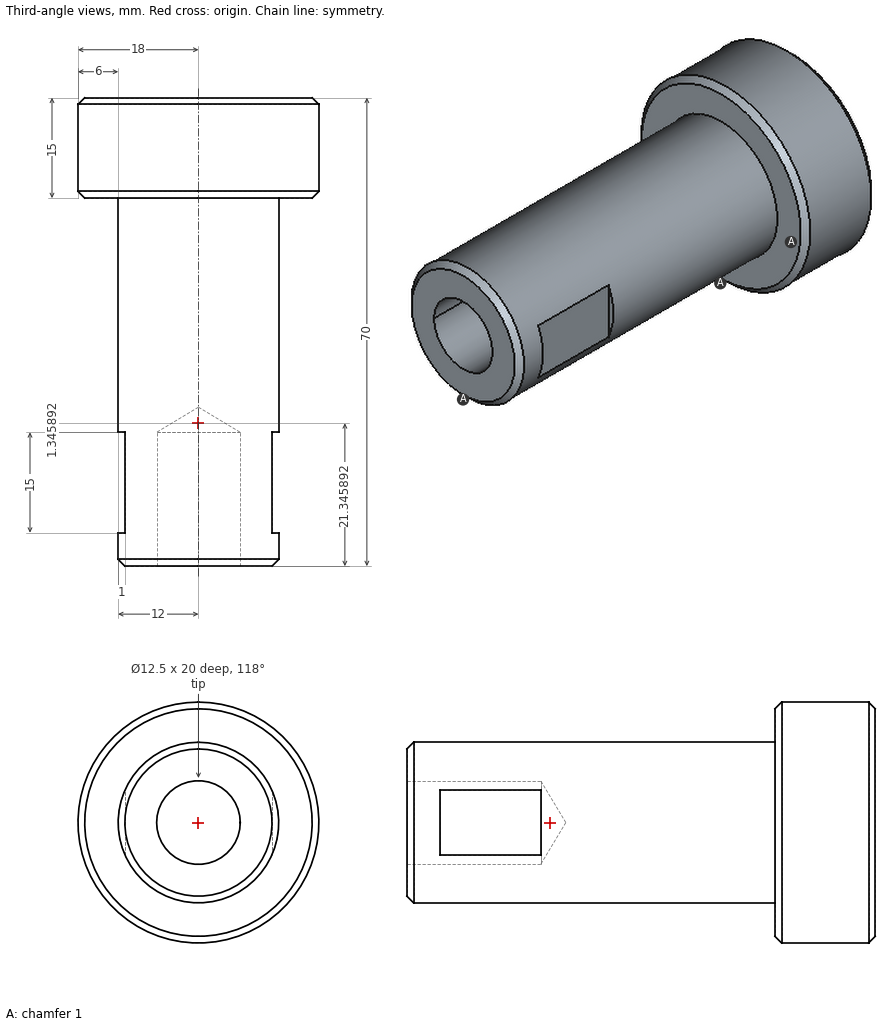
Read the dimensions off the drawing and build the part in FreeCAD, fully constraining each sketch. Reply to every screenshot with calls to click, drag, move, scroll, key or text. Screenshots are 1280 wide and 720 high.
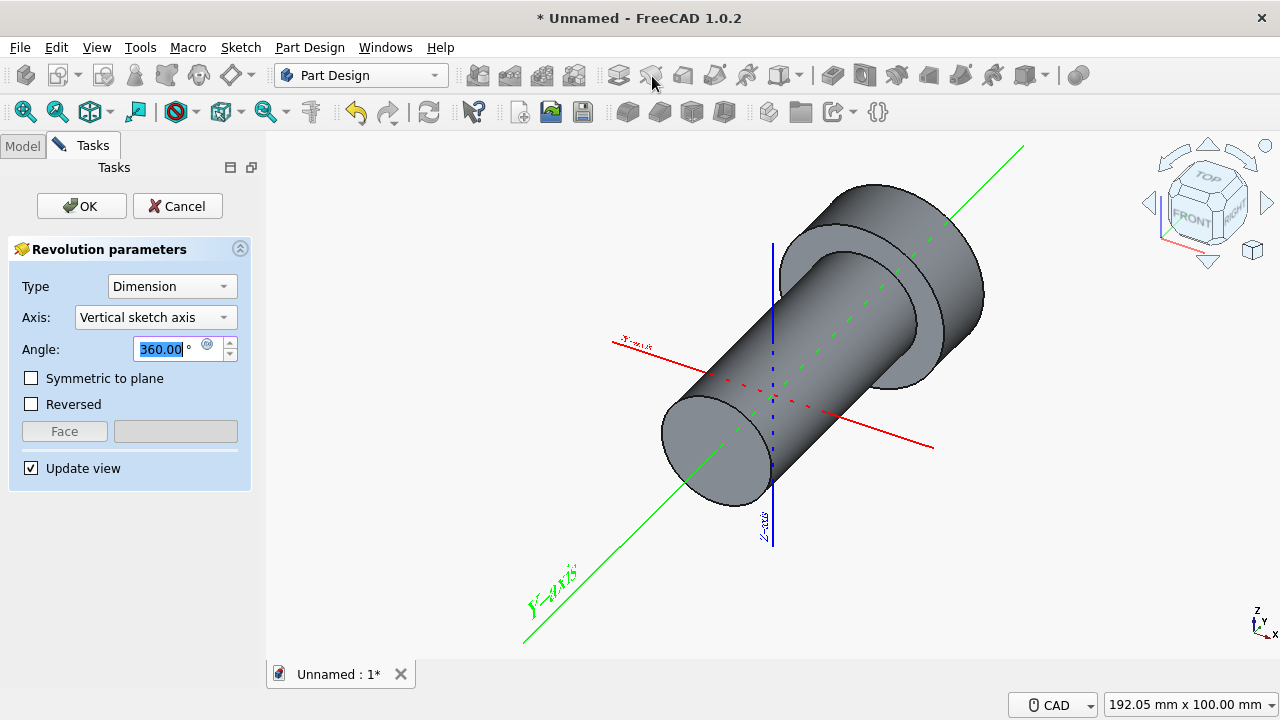
click(82, 206)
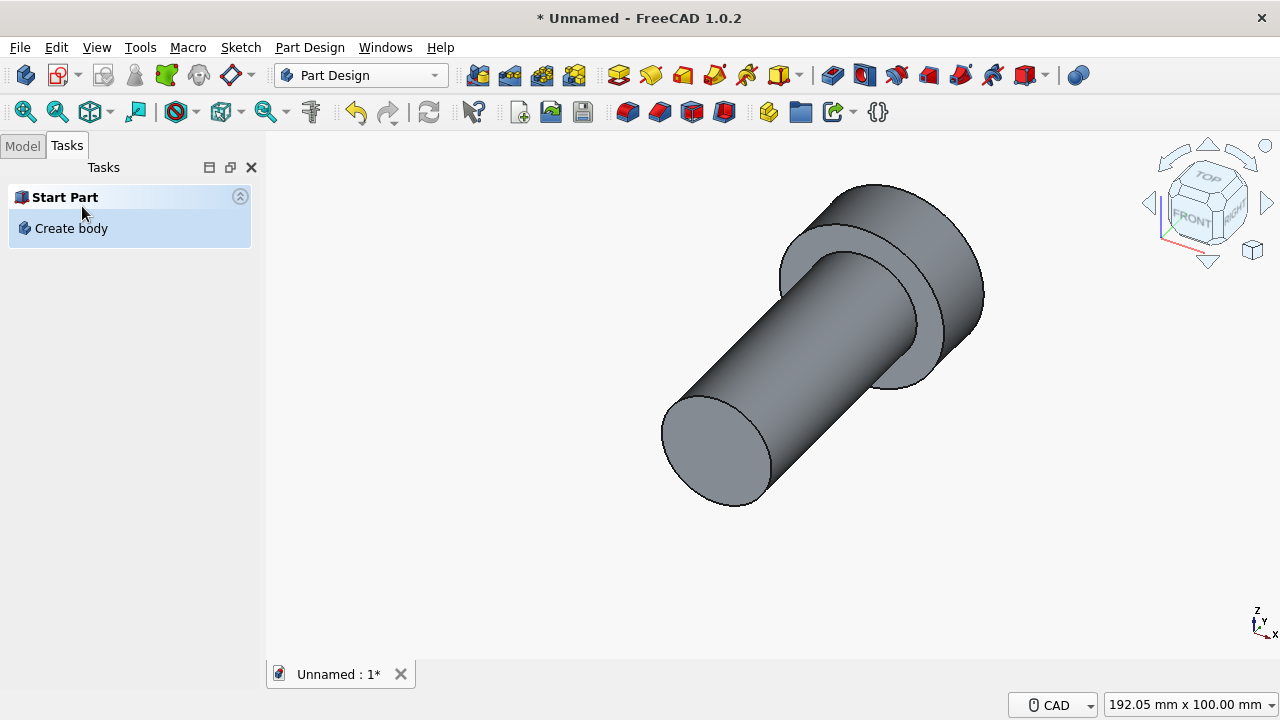
click(772, 468)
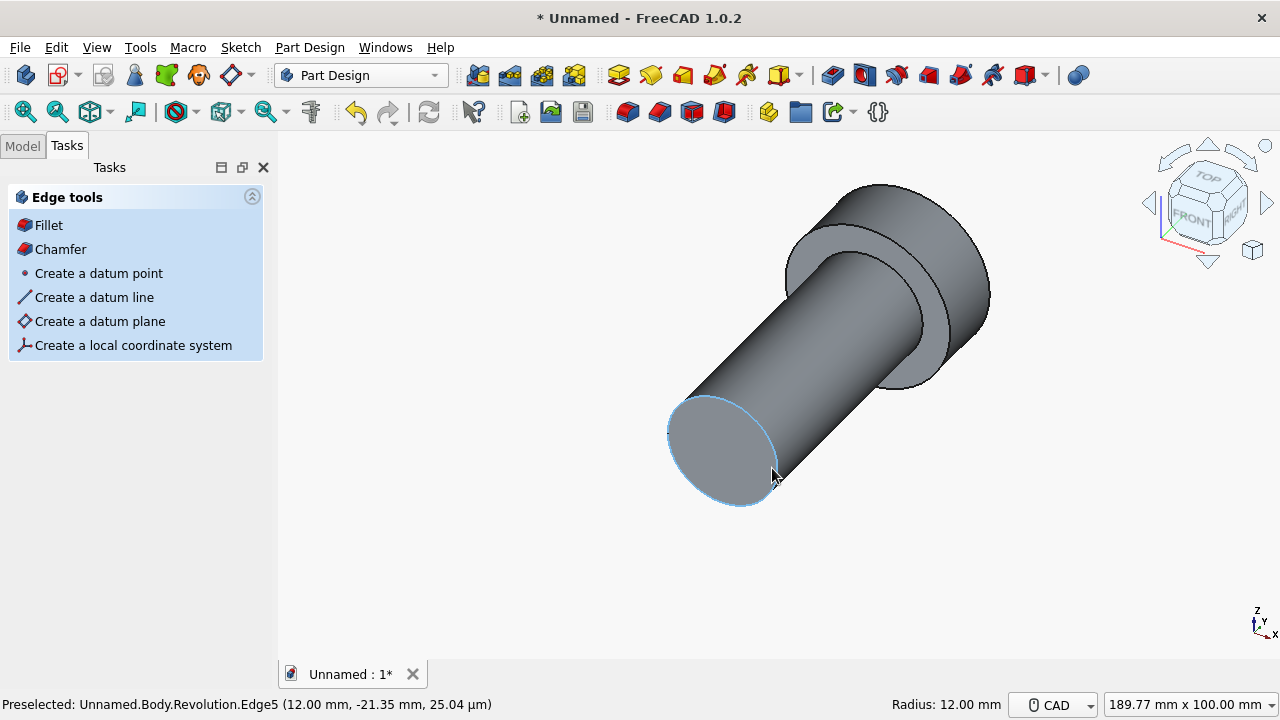
click(950, 333, ctrl)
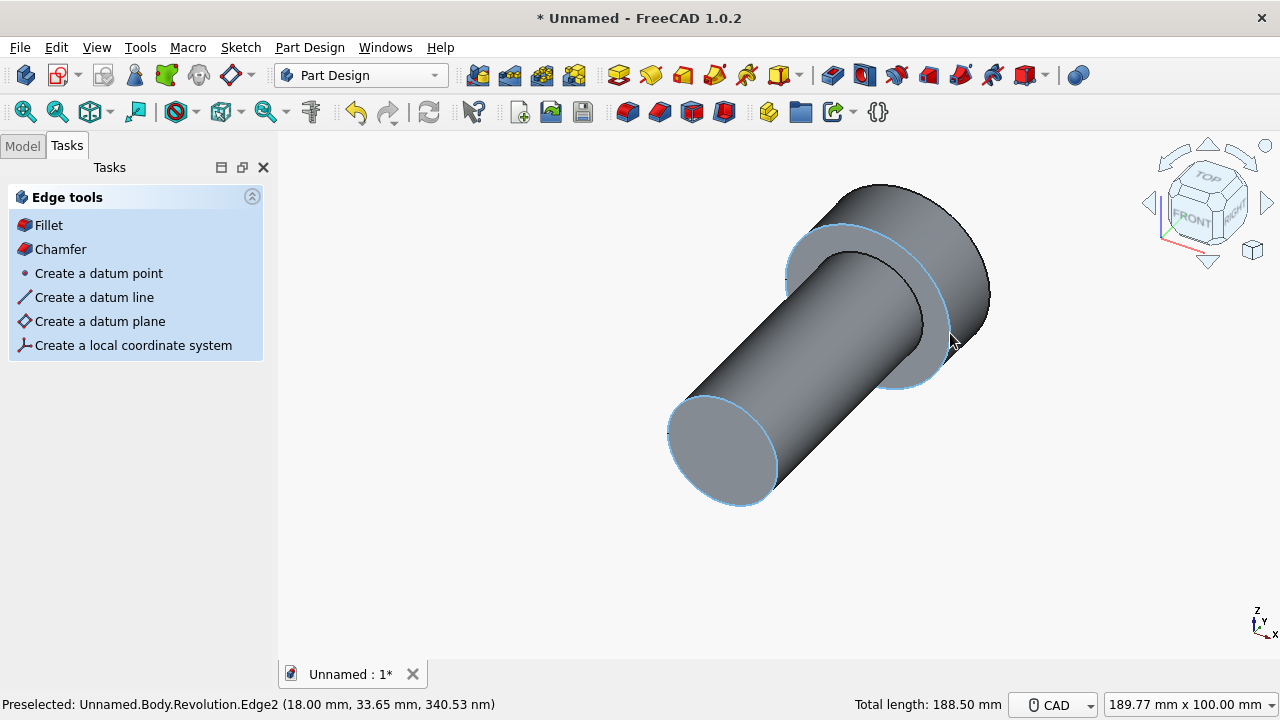
key(0)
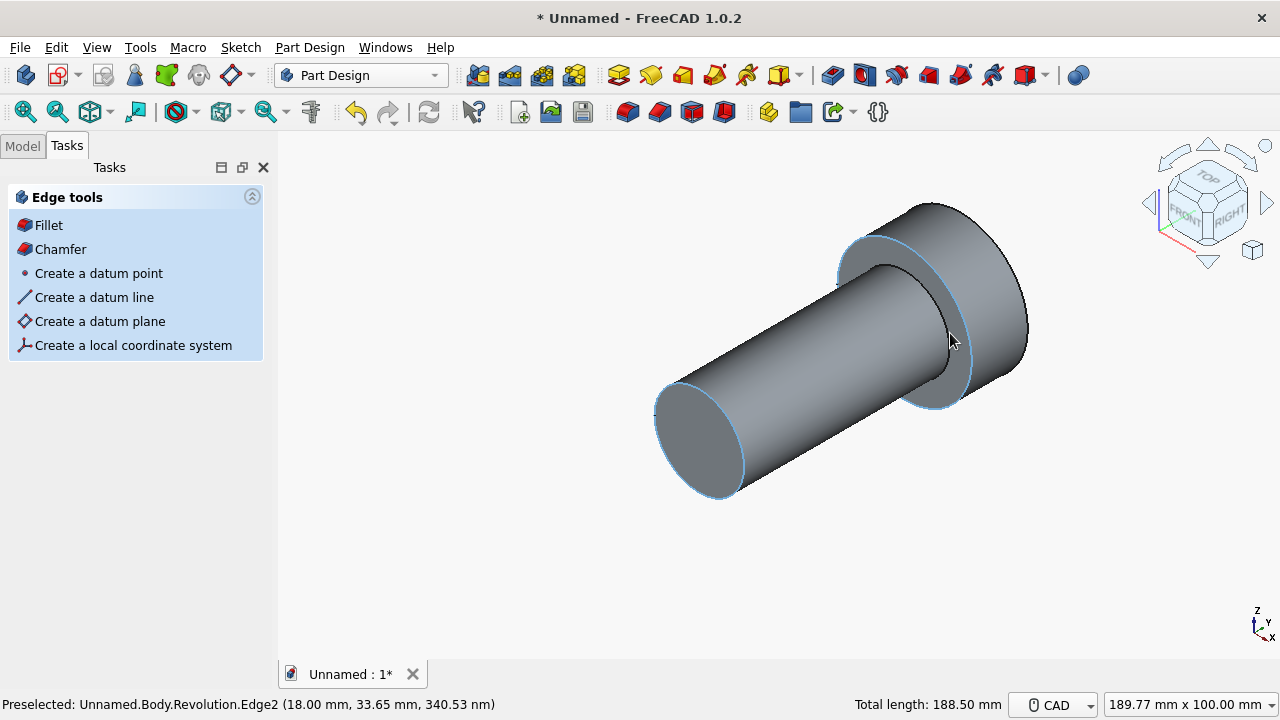
key(2)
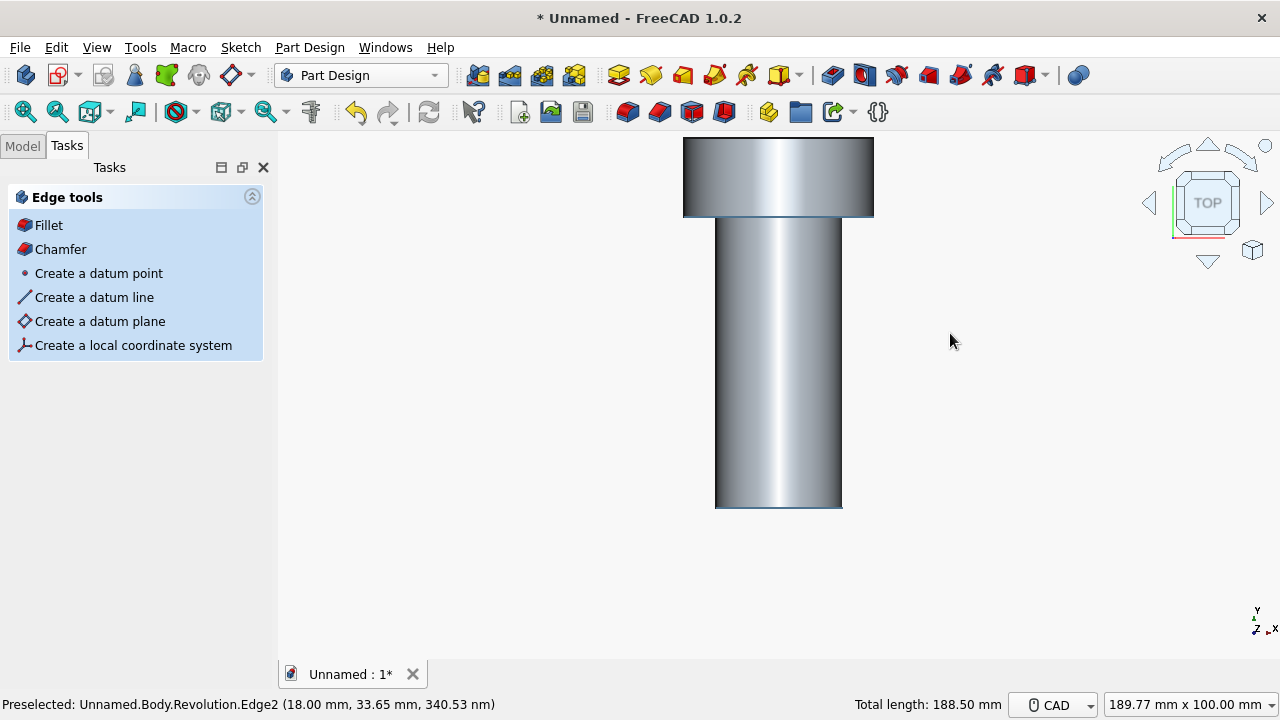
key(1)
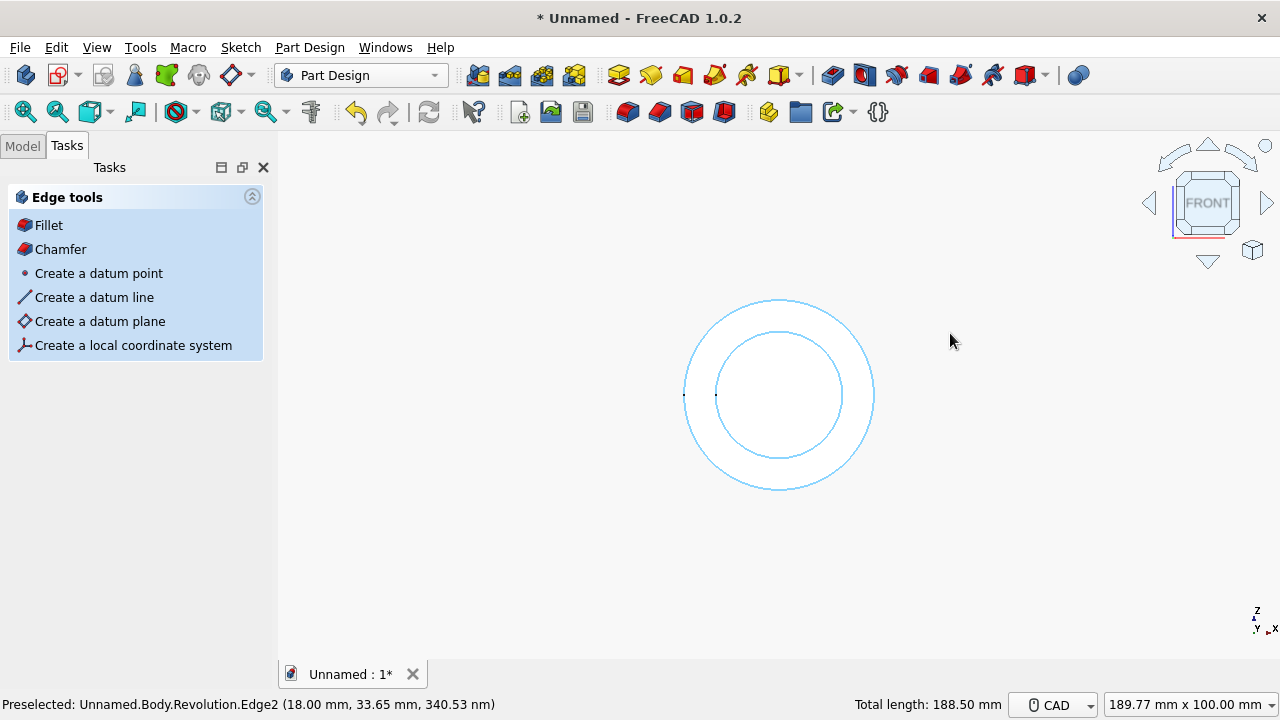
click(26, 112)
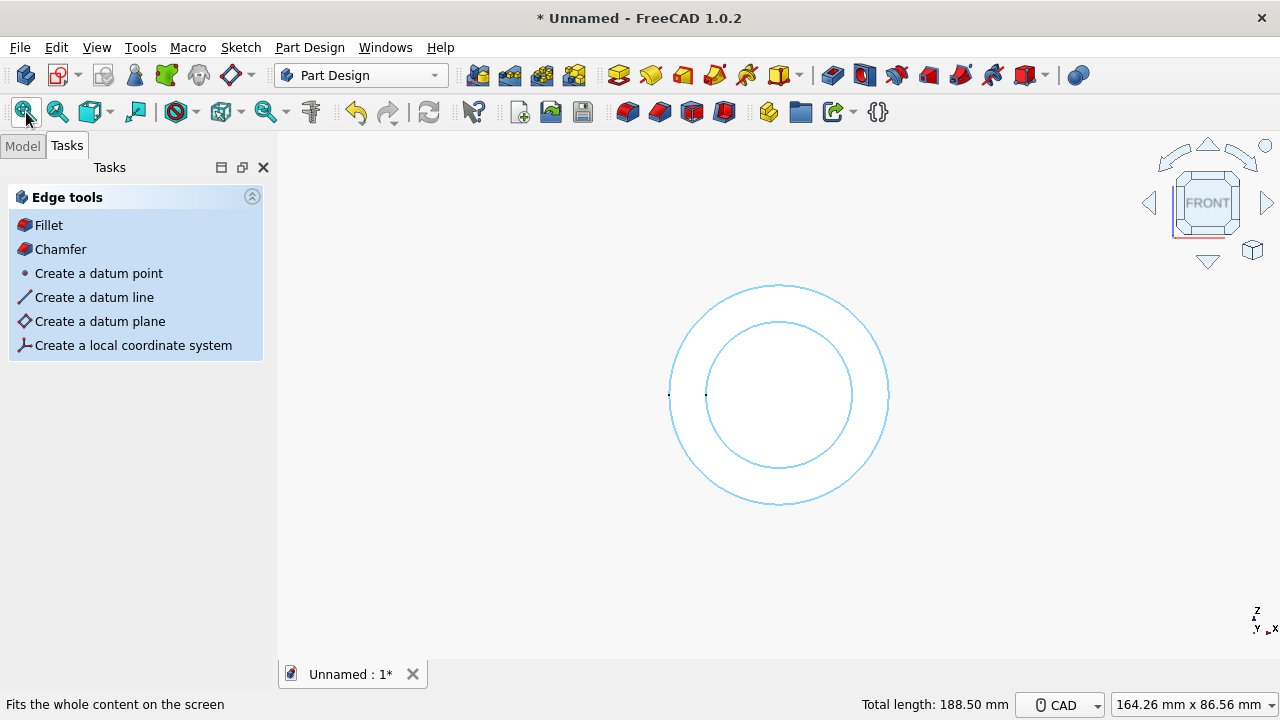
key(3)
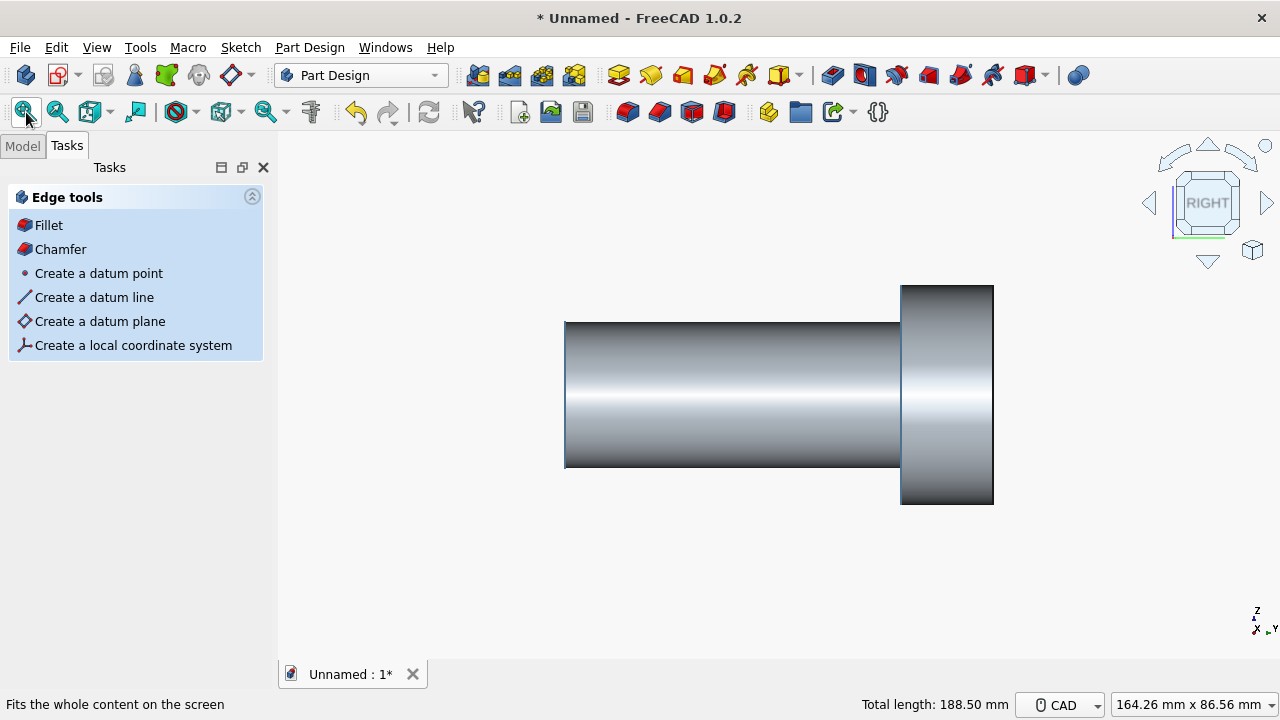
click(26, 112)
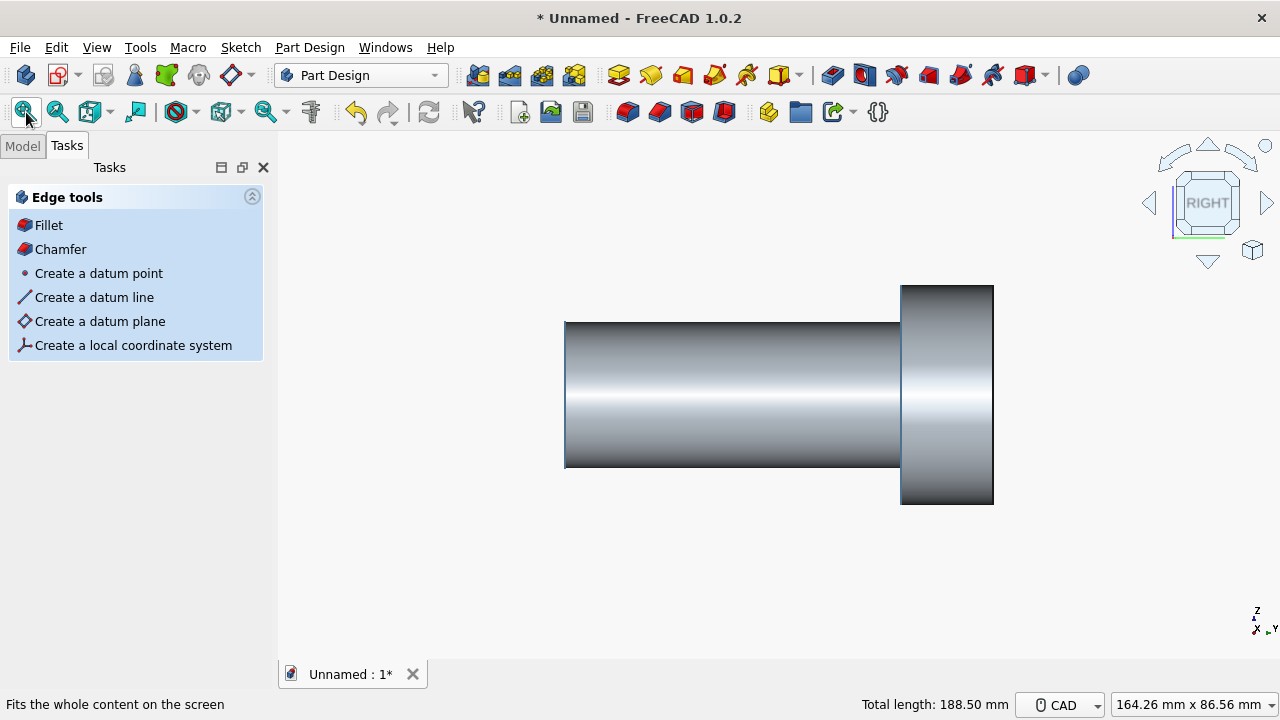
click(993, 394, ctrl)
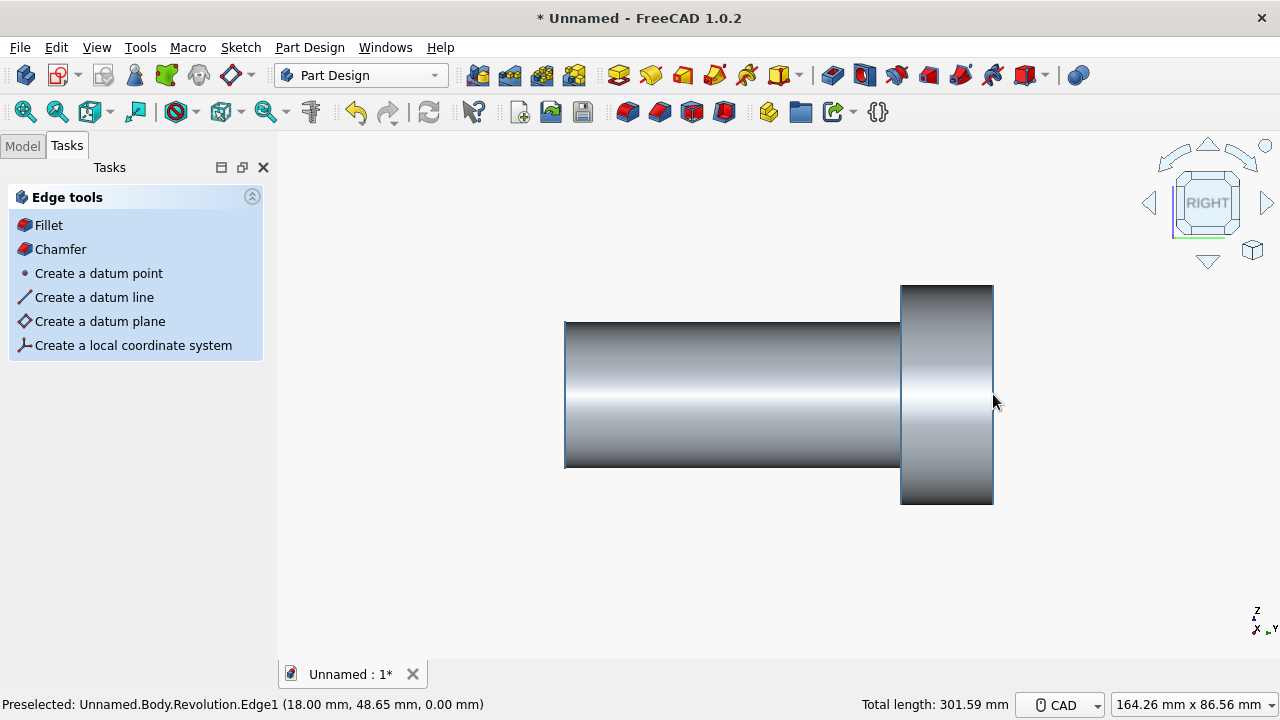
click(660, 112)